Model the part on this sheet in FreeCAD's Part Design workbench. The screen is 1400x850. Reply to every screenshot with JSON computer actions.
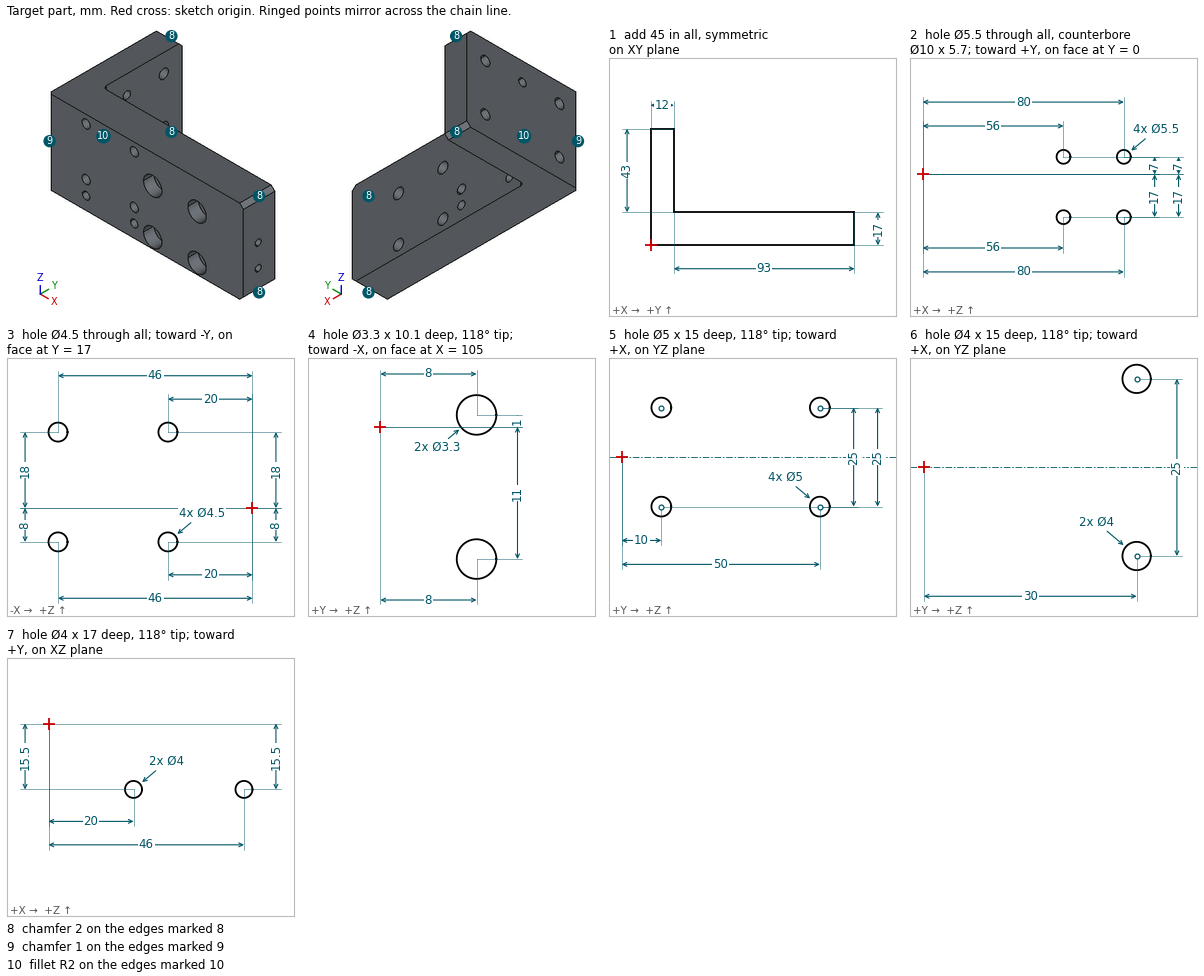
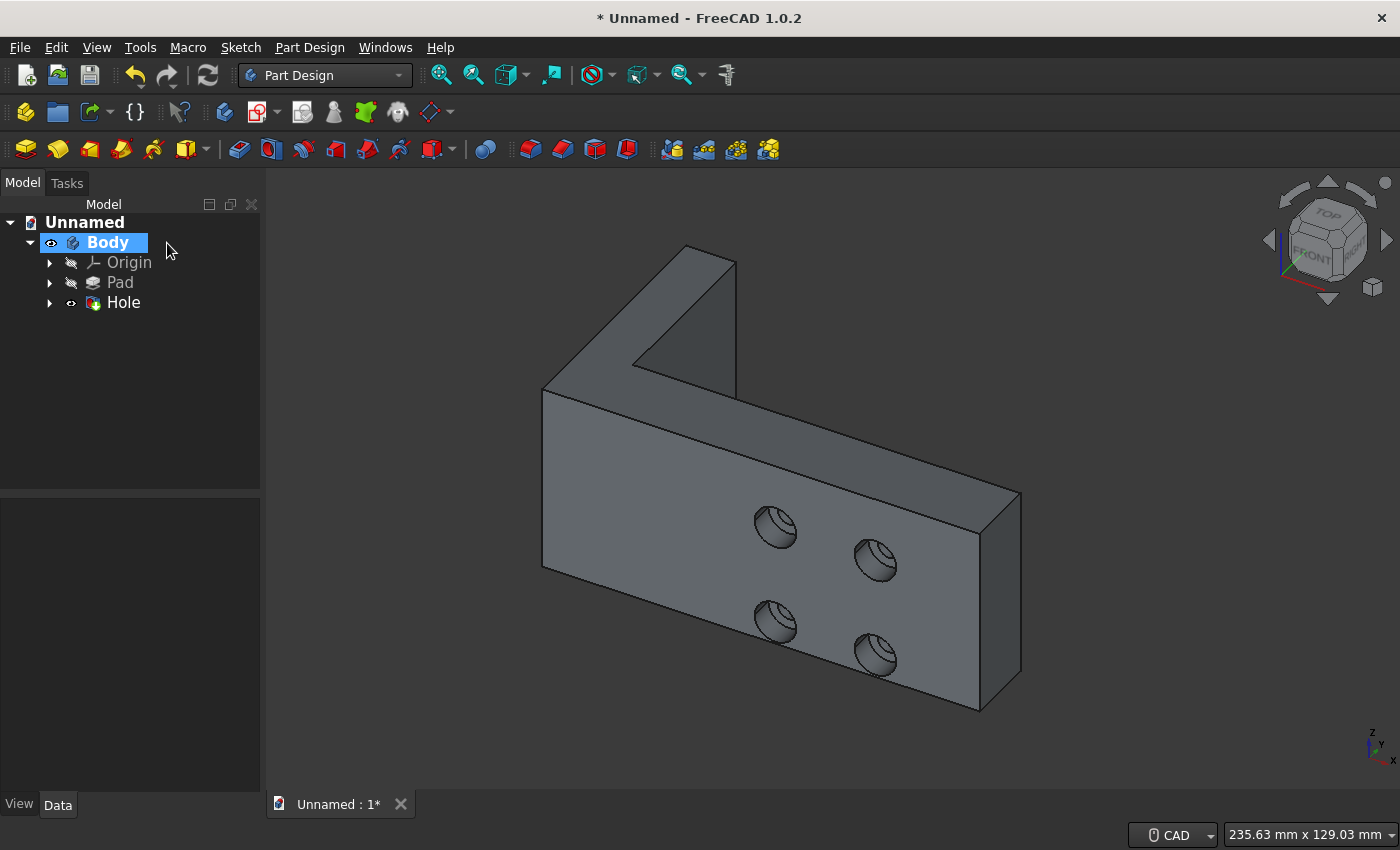
{"action": "key", "text": "4"}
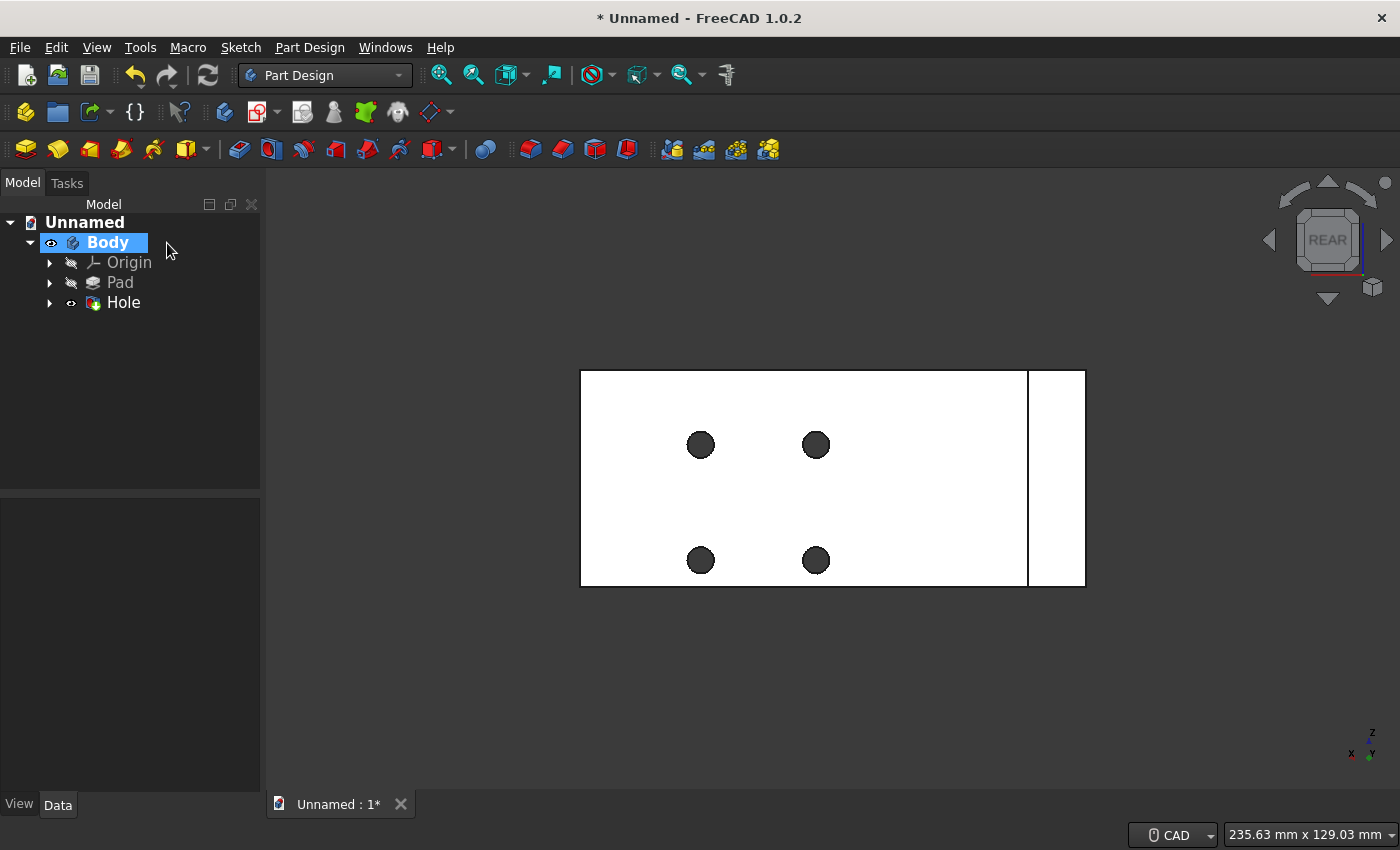
{"action": "left_click", "coordinate": [442, 76]}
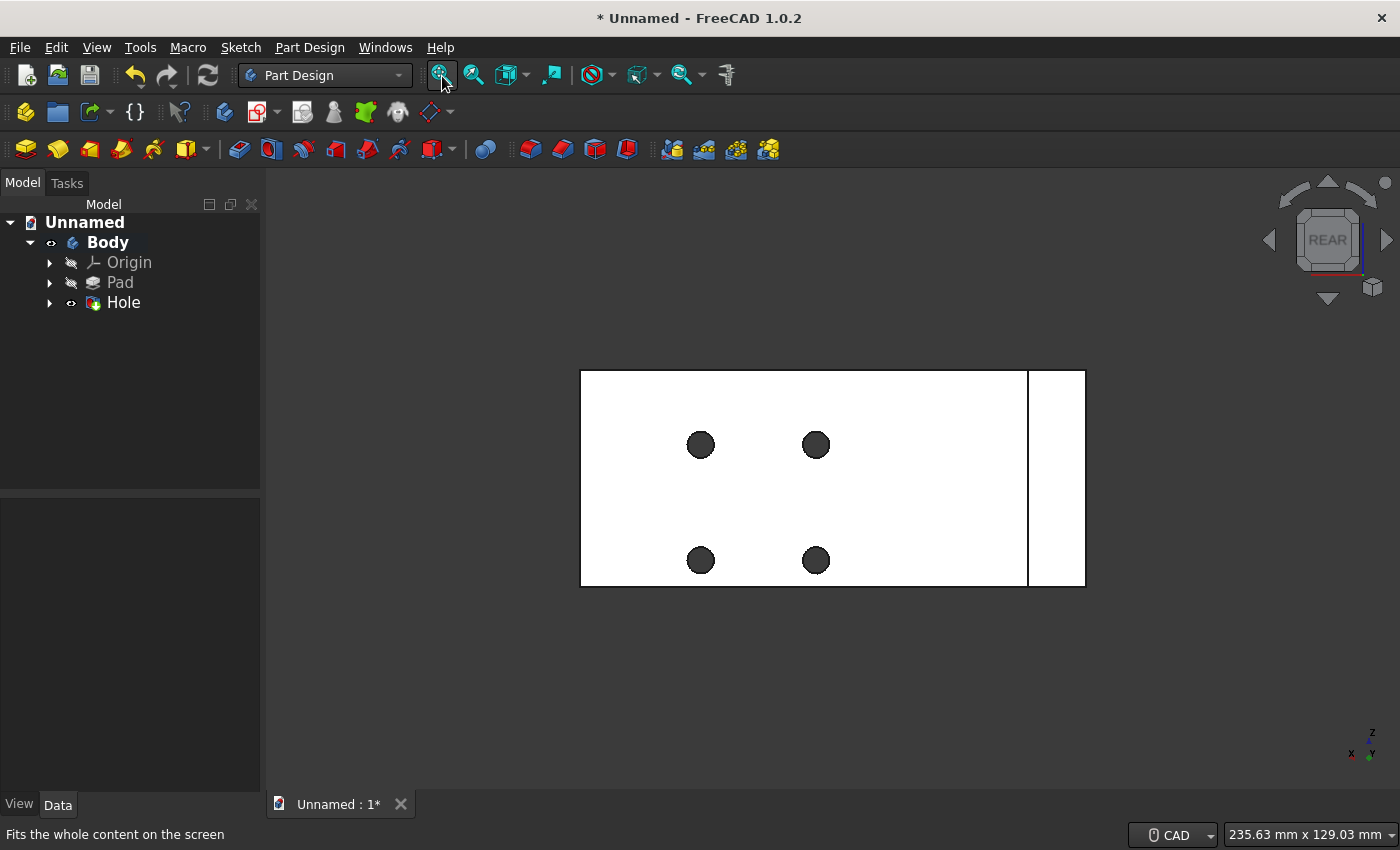
{"action": "left_click", "coordinate": [932, 478]}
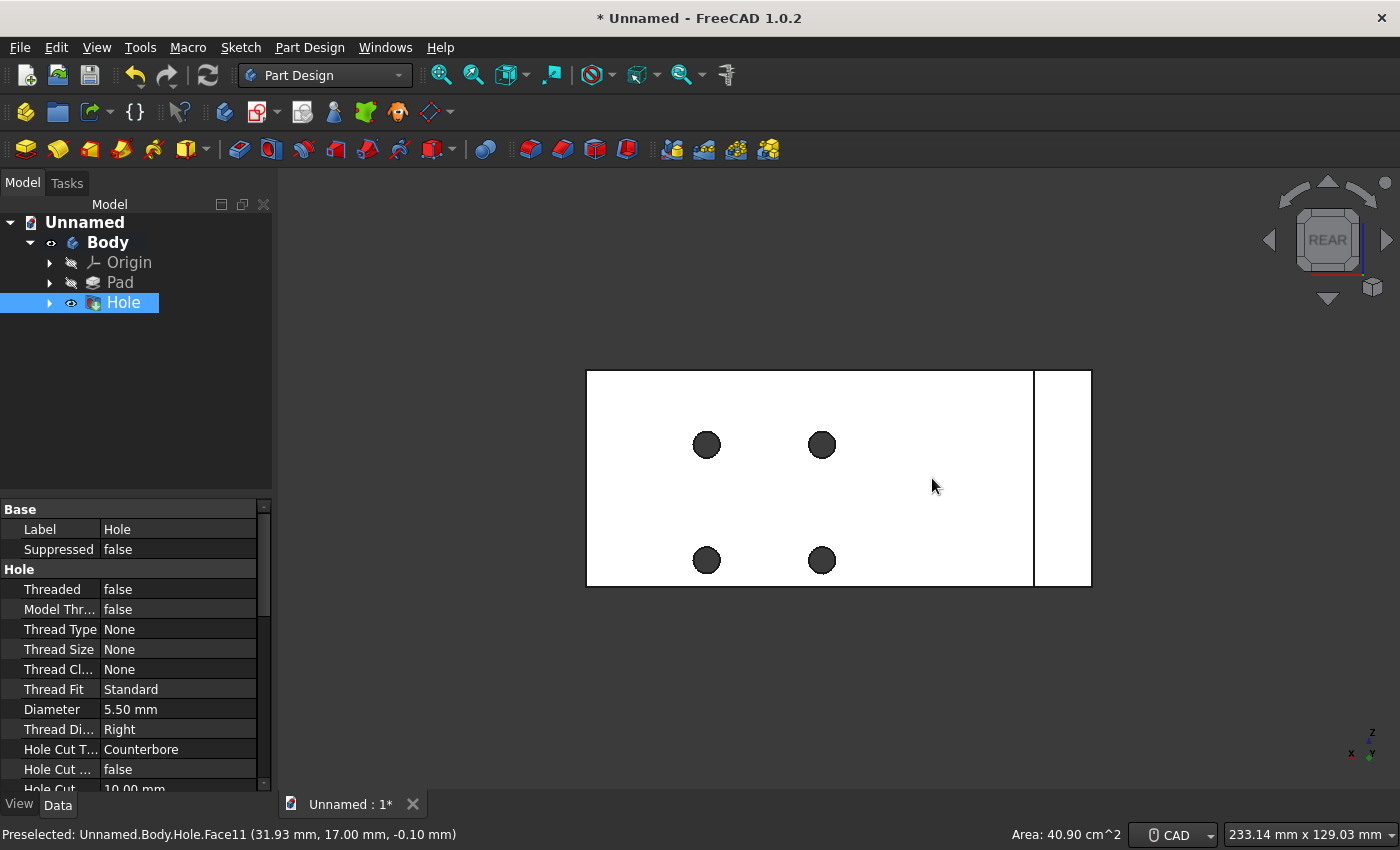
{"action": "left_click", "coordinate": [258, 112]}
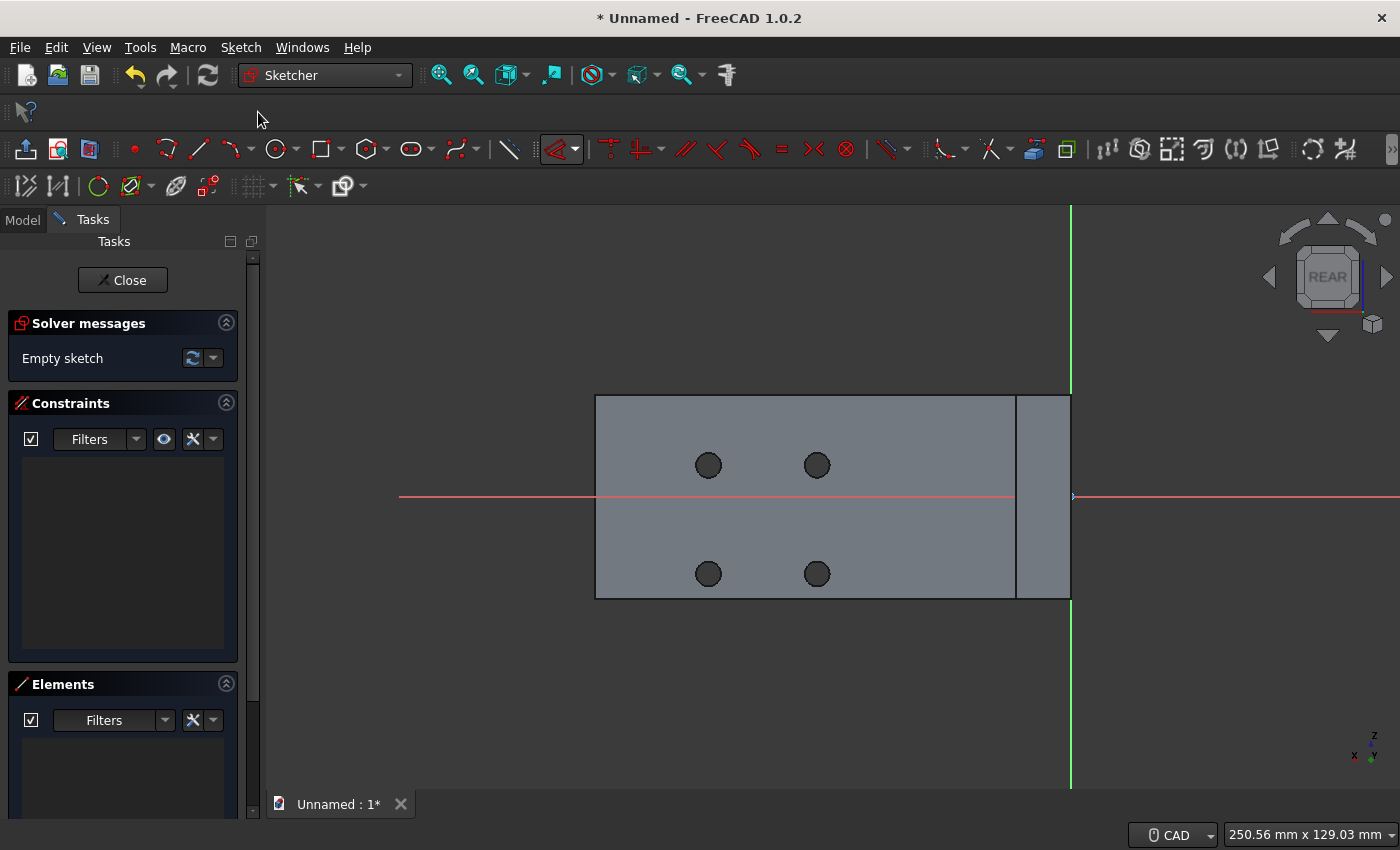
{"action": "key", "text": "q s"}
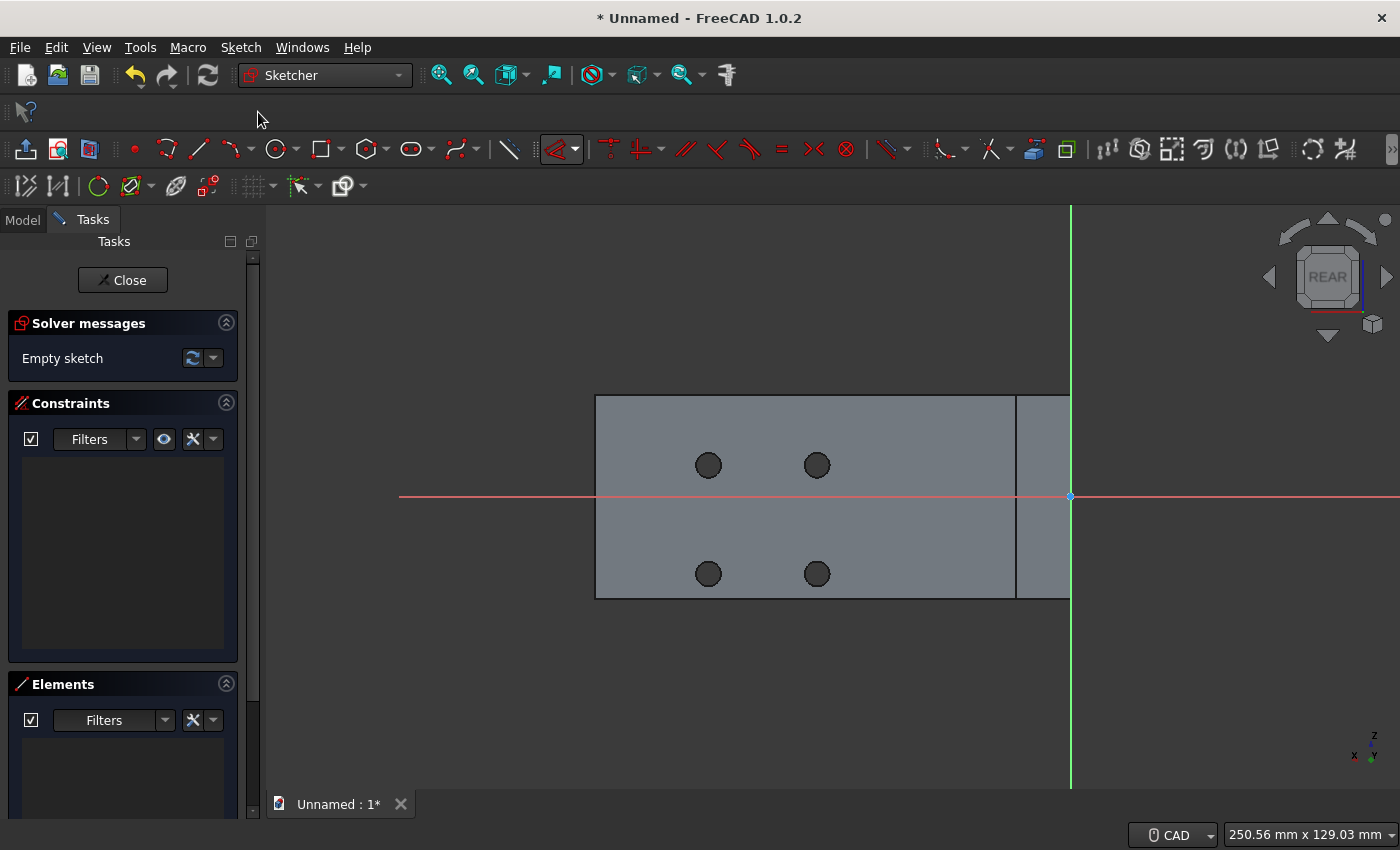
{"action": "scroll", "coordinate": [1076, 461], "scroll_direction": "up", "scroll_amount": 5}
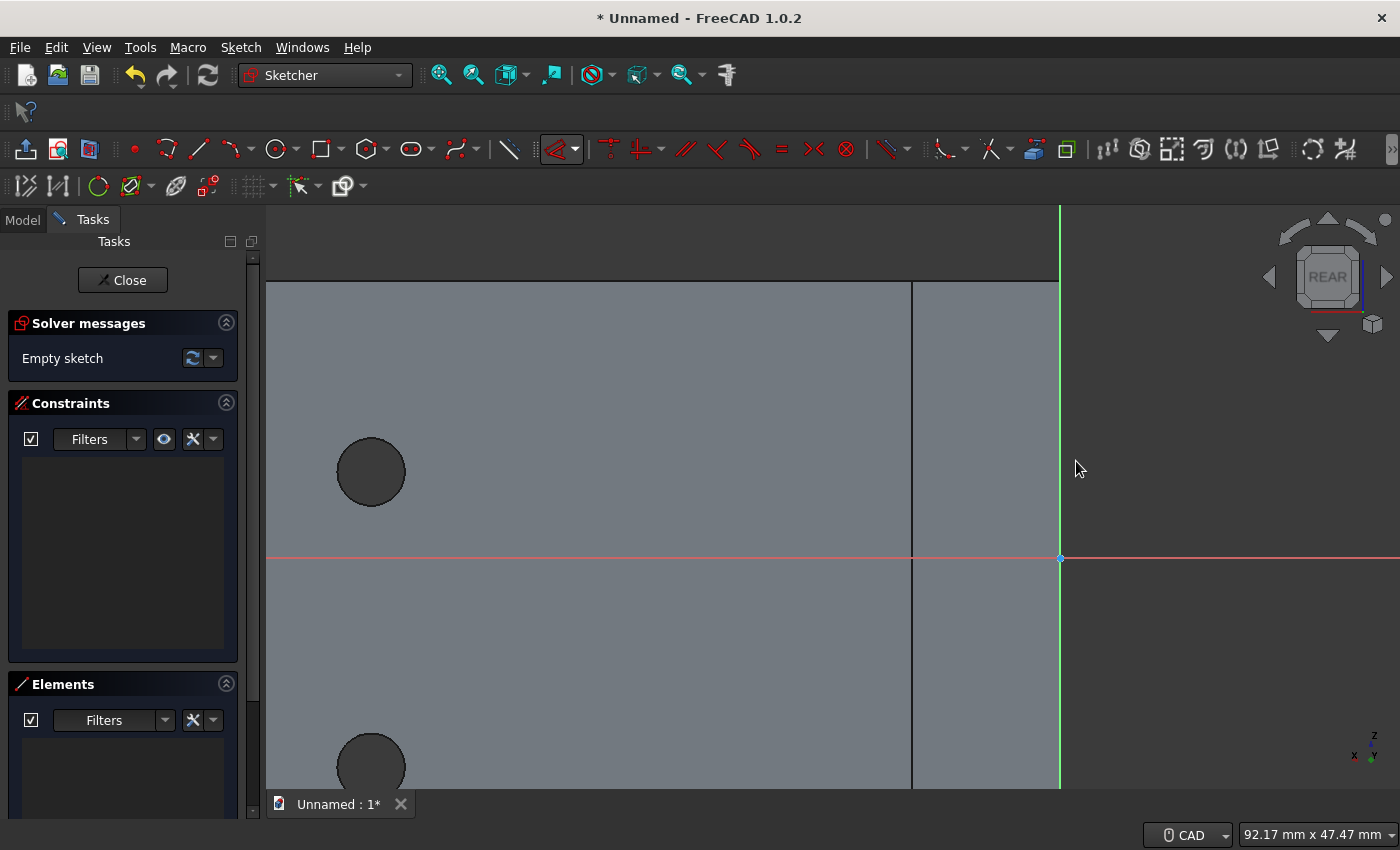
{"action": "key", "text": "g c"}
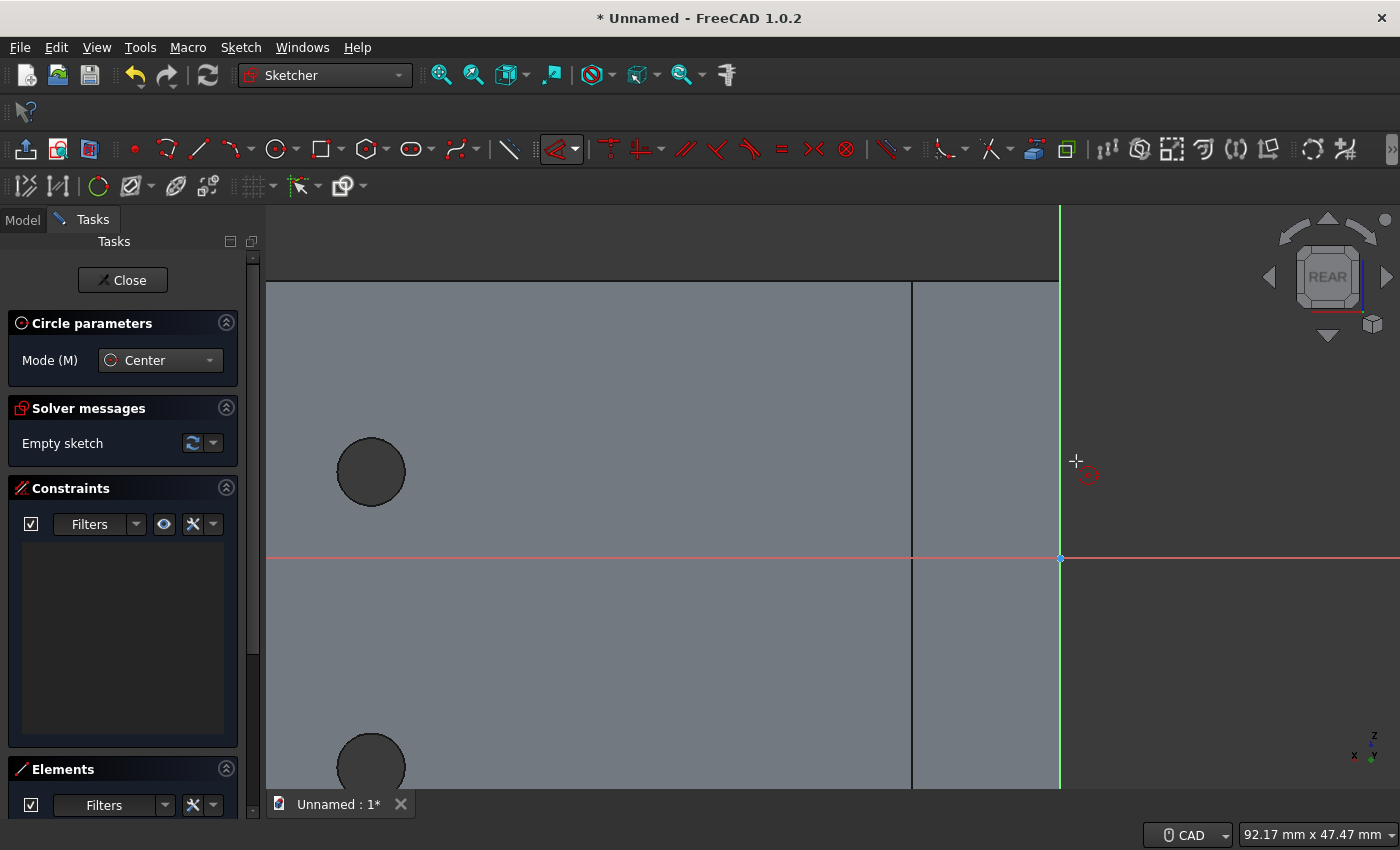
{"action": "left_click", "coordinate": [814, 657]}
{"action": "left_click", "coordinate": [834, 637]}